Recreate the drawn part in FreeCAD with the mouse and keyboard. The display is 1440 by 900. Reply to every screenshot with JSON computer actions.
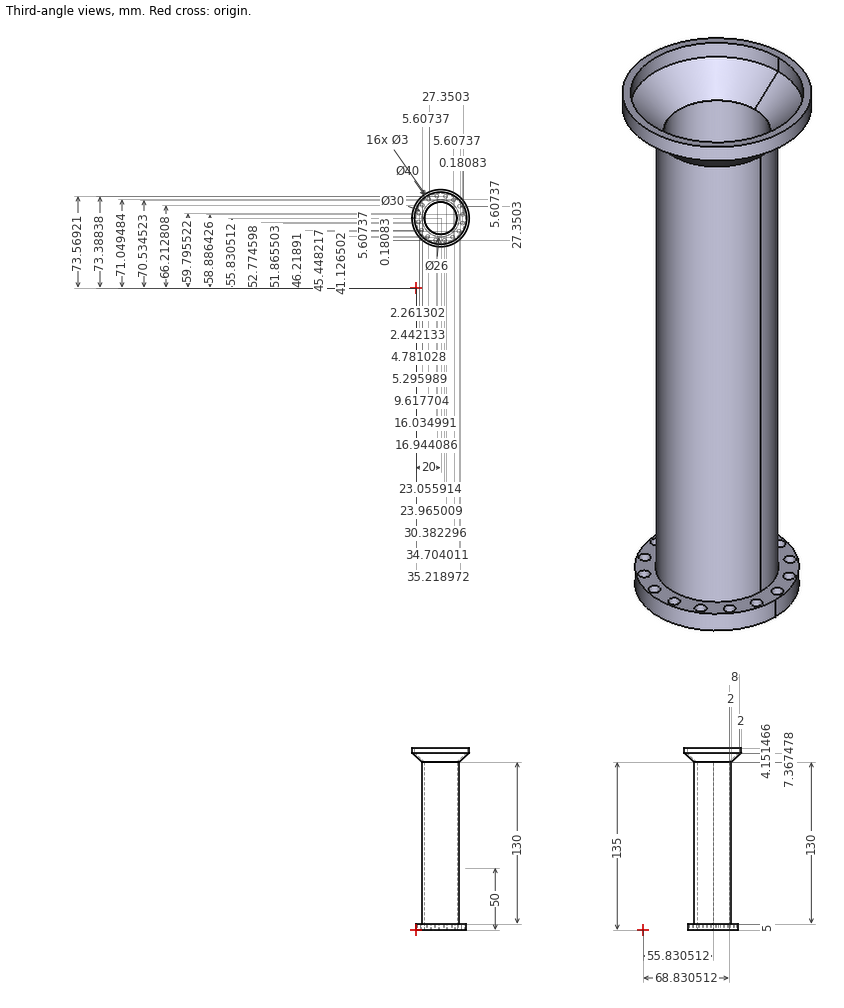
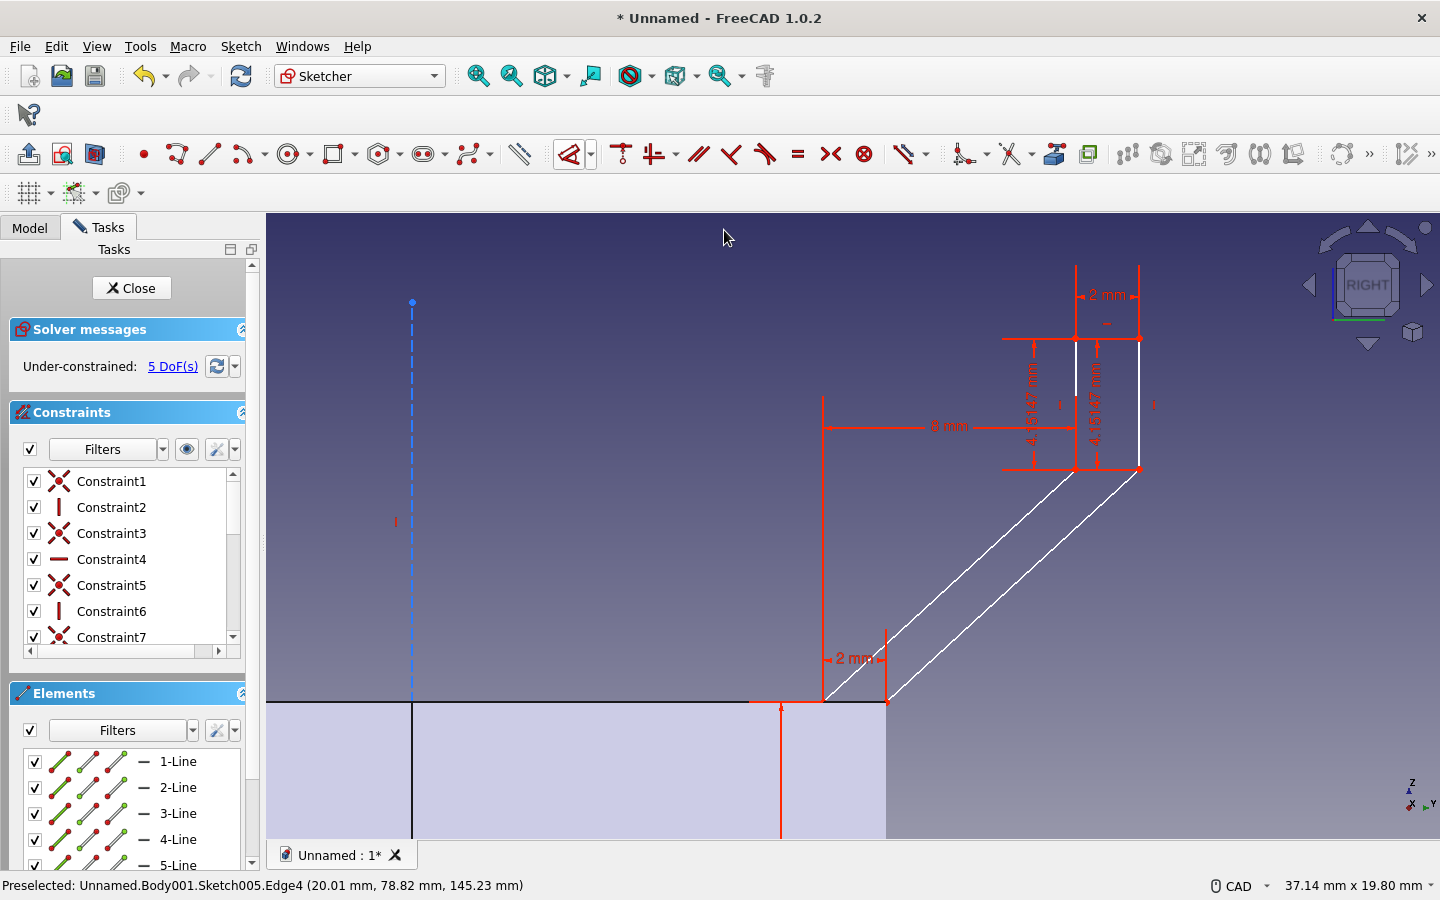
{"action": "left_click", "coordinate": [899, 633]}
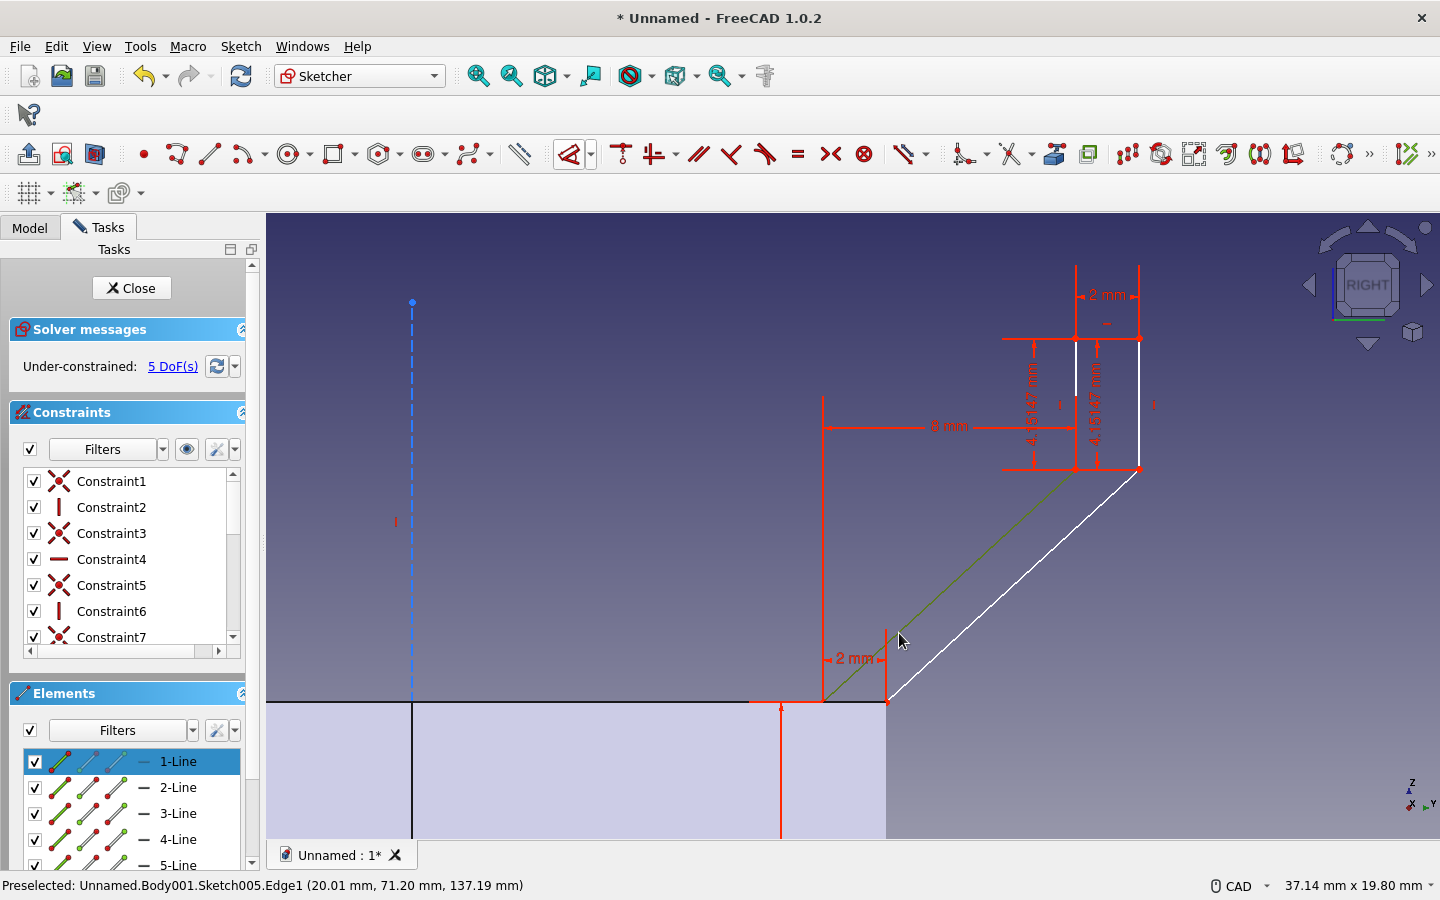
{"action": "left_click", "coordinate": [590, 154]}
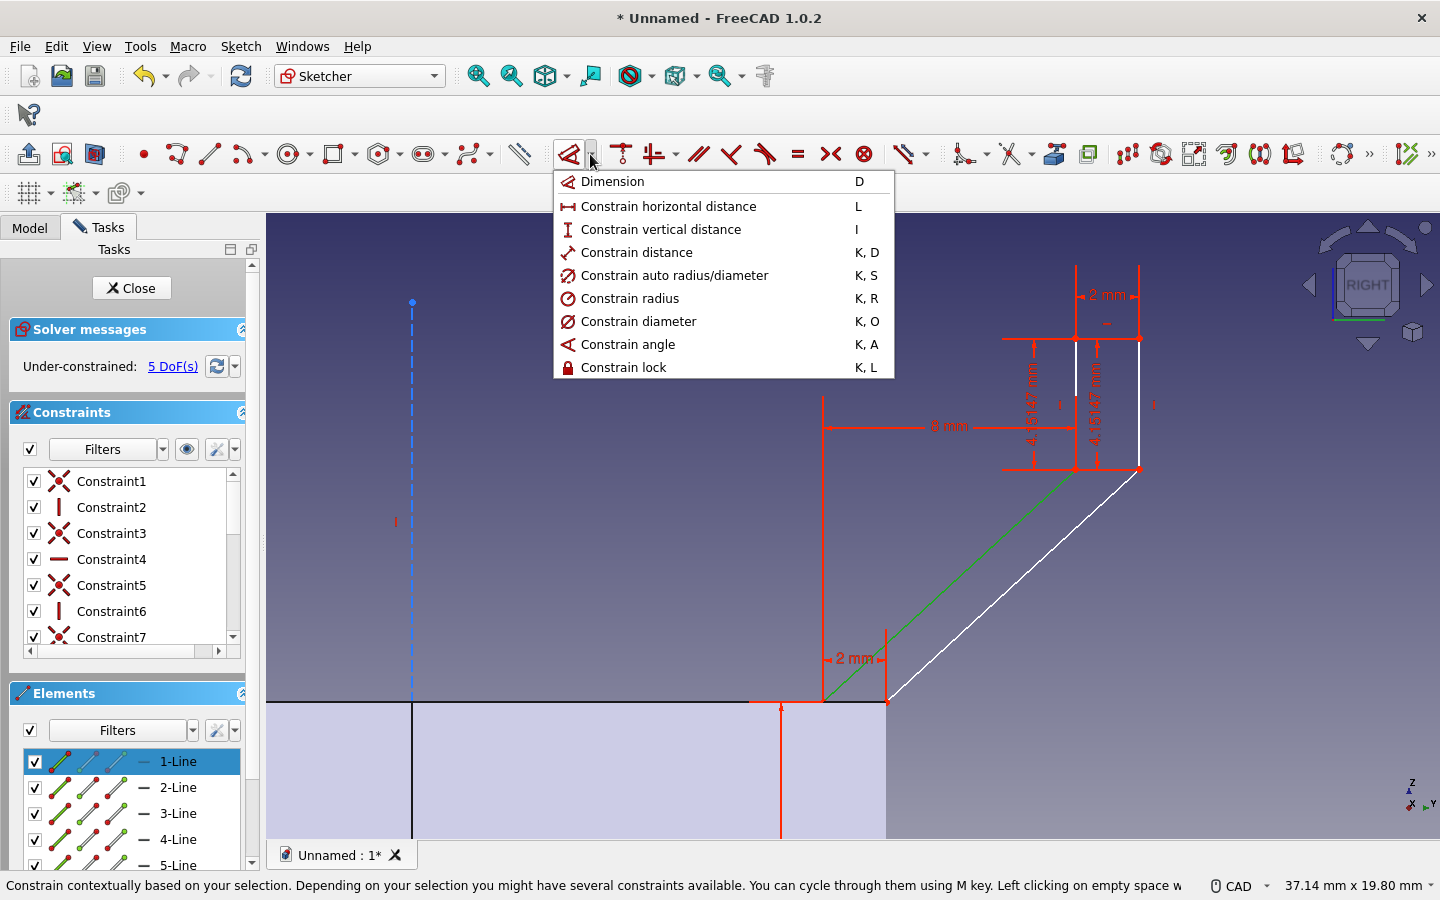
{"action": "left_click", "coordinate": [724, 230]}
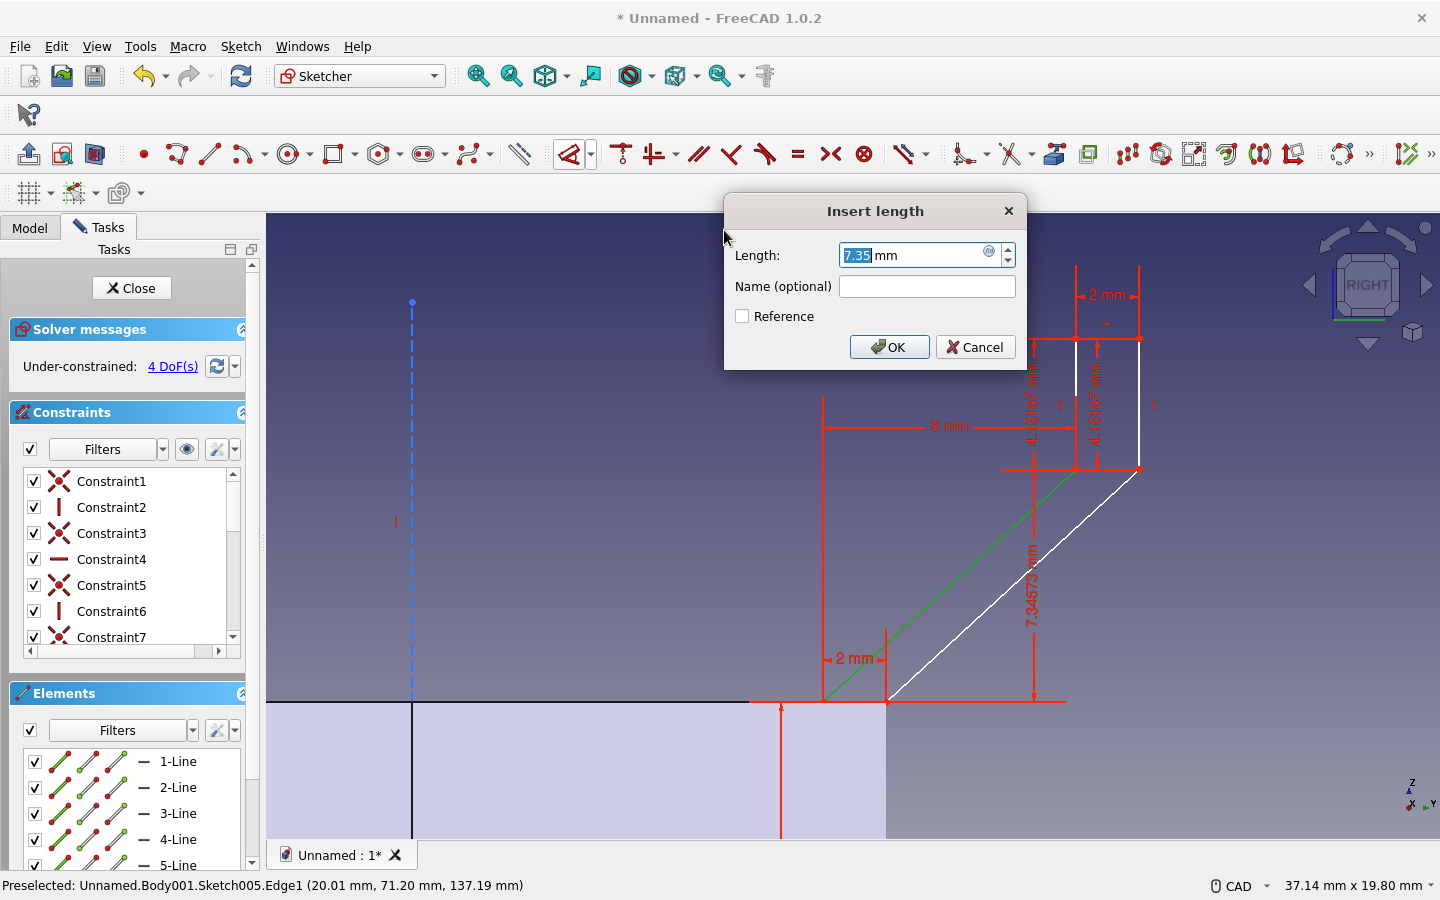
{"action": "type", "text": "7.367478"}
{"action": "key", "text": "Return"}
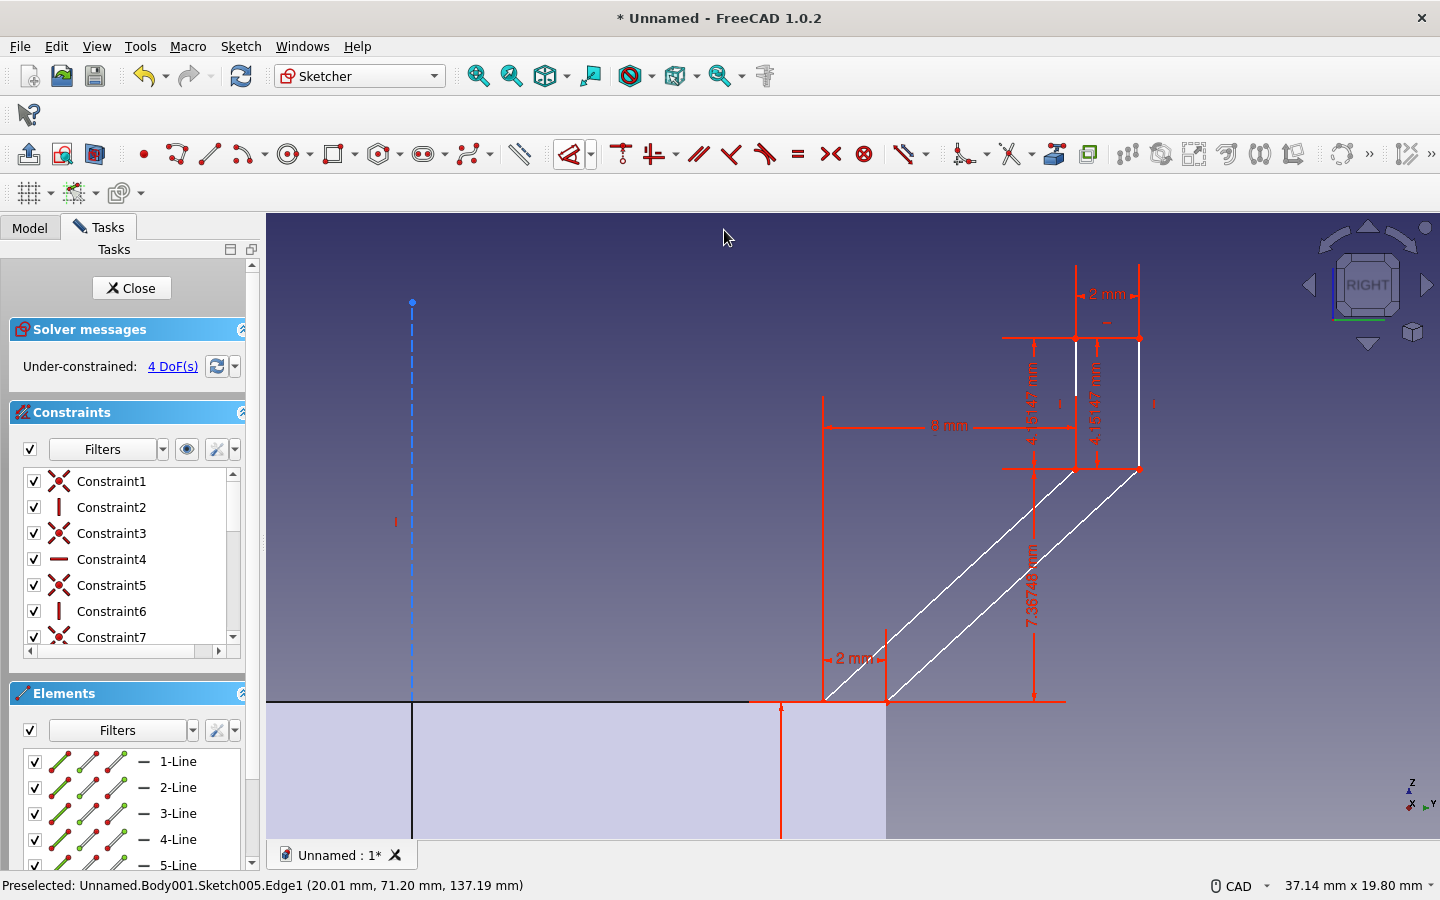
{"action": "left_click", "coordinate": [823, 702]}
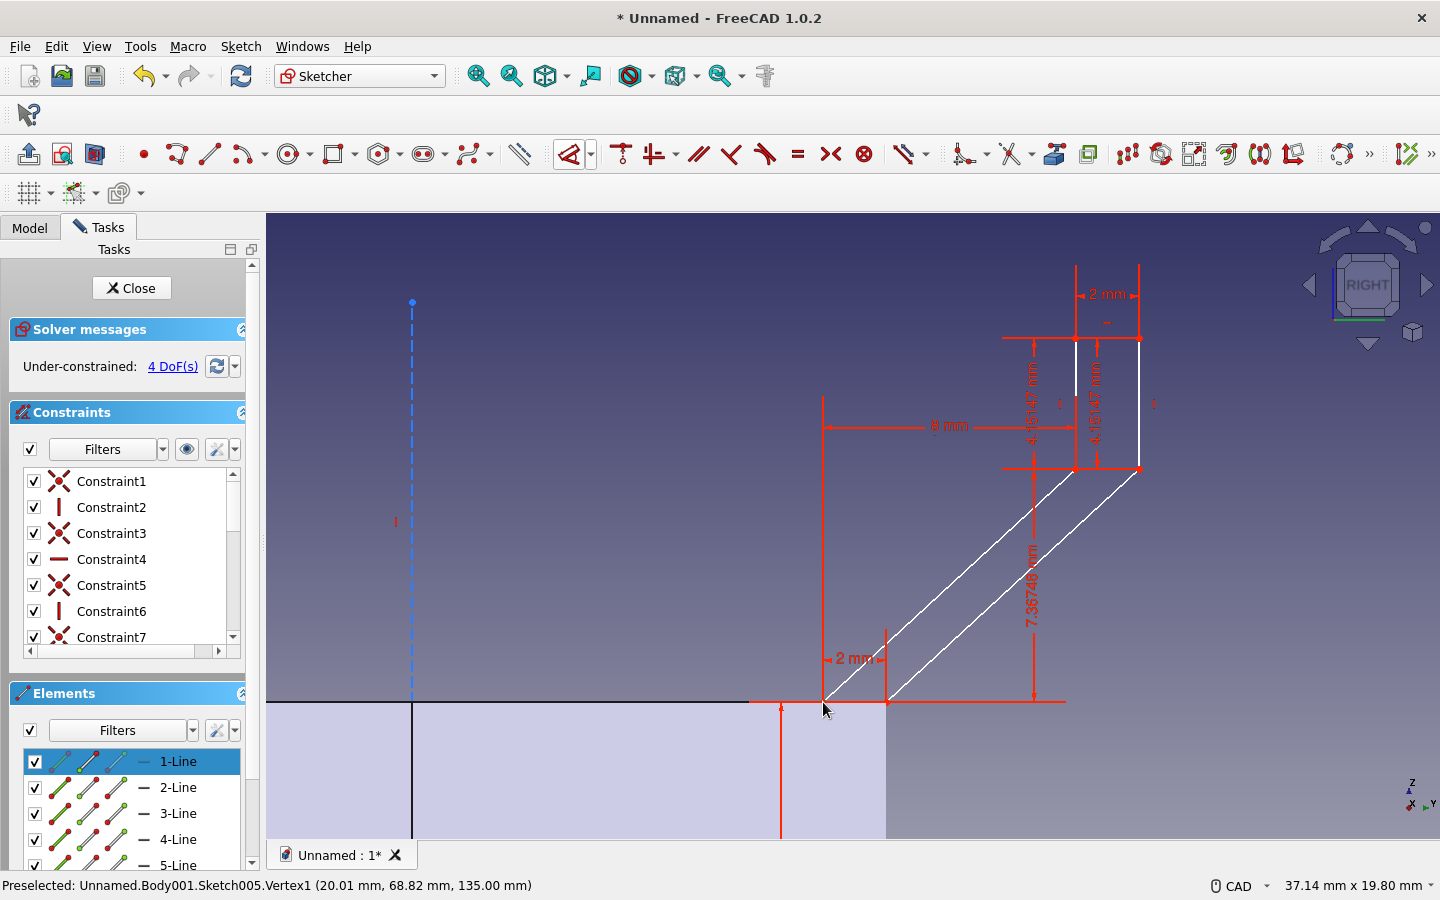
{"action": "key", "text": "l"}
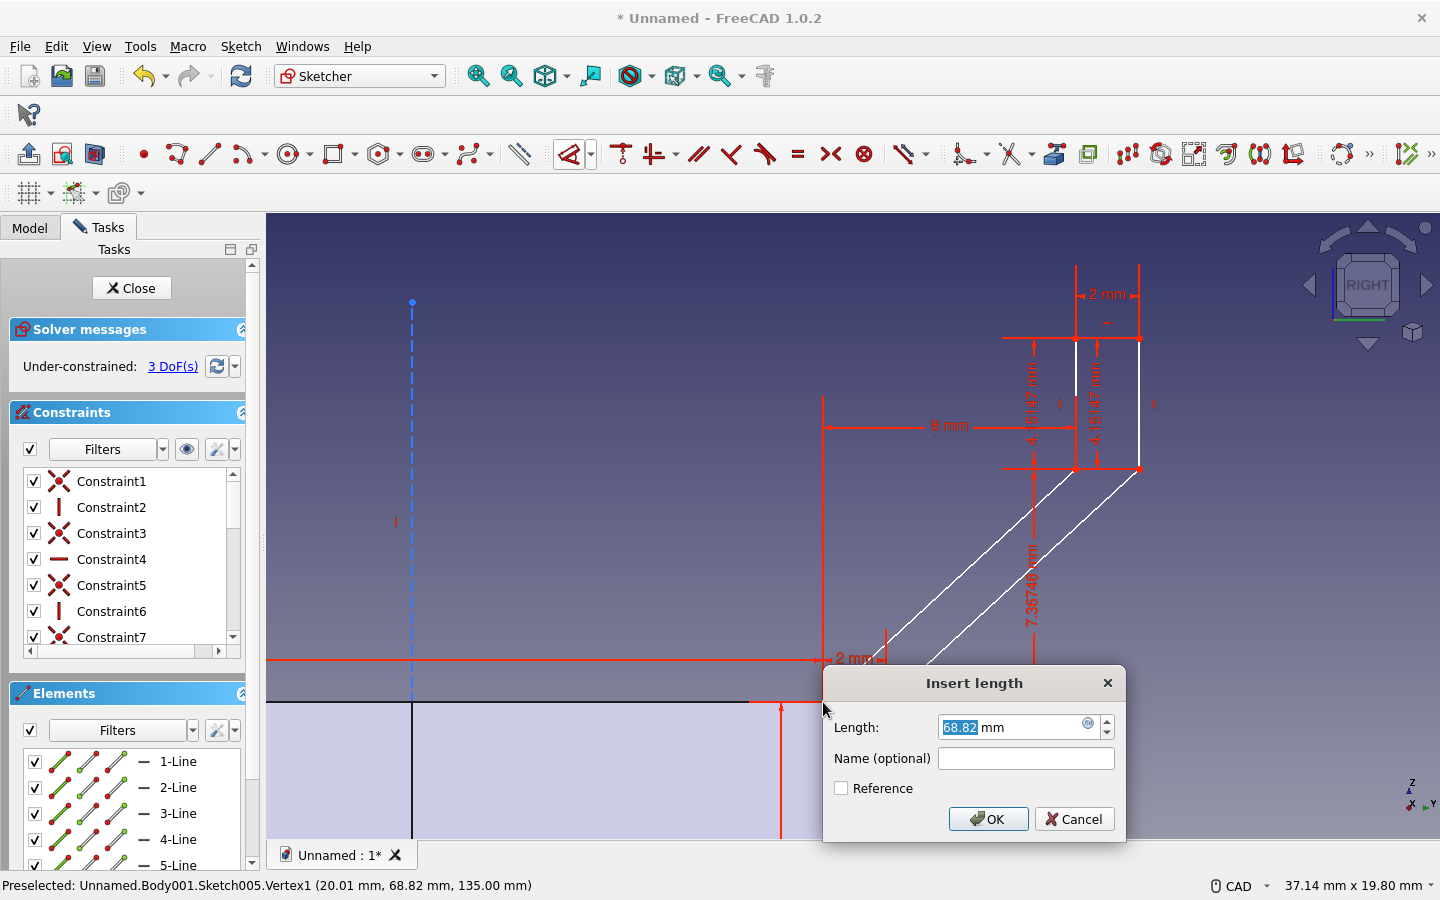
{"action": "type", "text": "68.830512"}
{"action": "key", "text": "Return"}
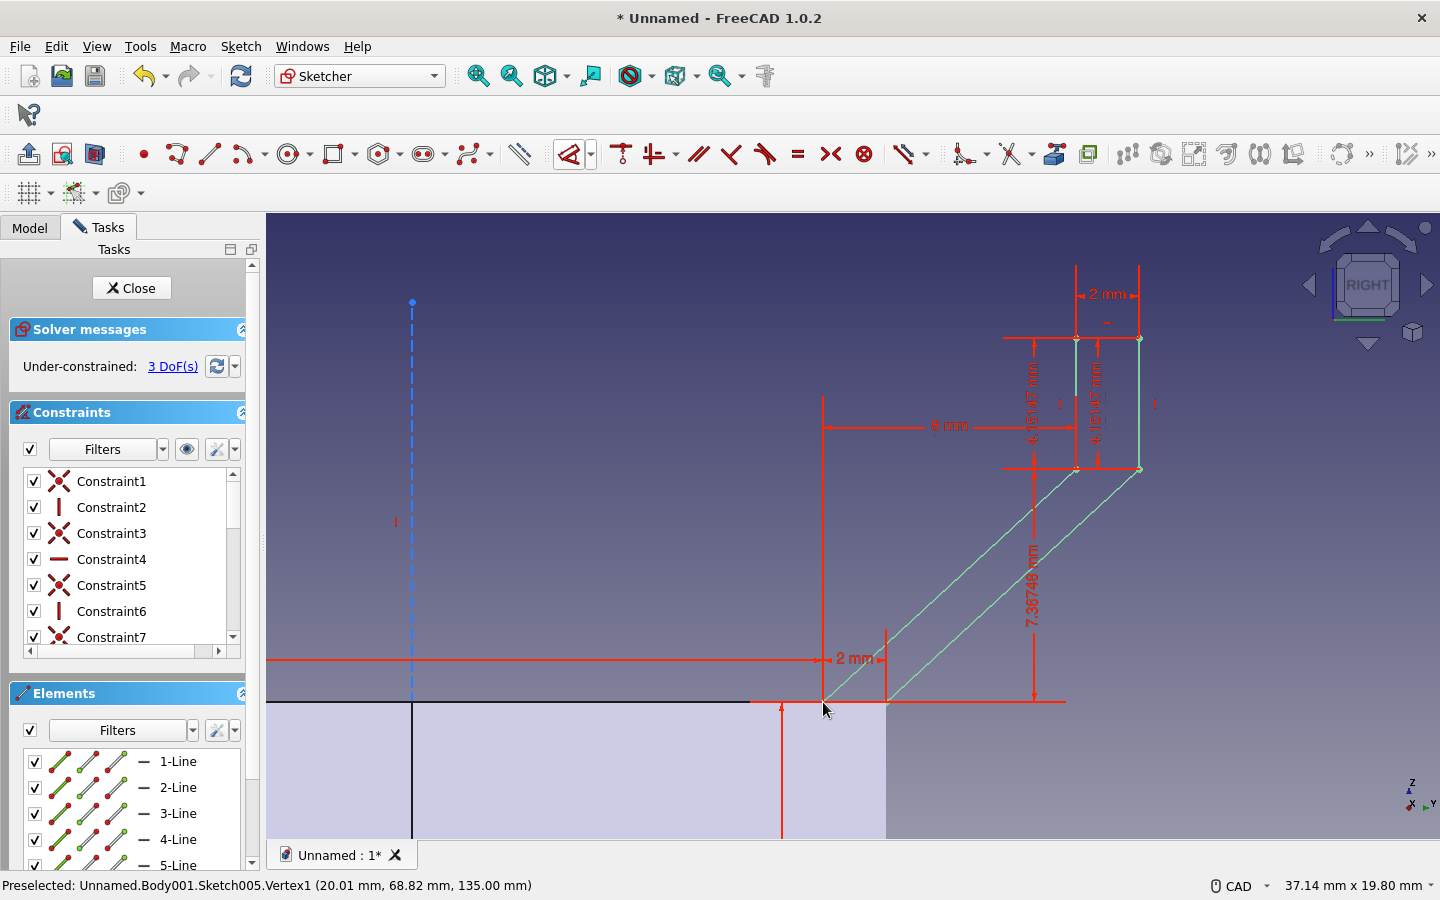
{"action": "left_click", "coordinate": [412, 740]}